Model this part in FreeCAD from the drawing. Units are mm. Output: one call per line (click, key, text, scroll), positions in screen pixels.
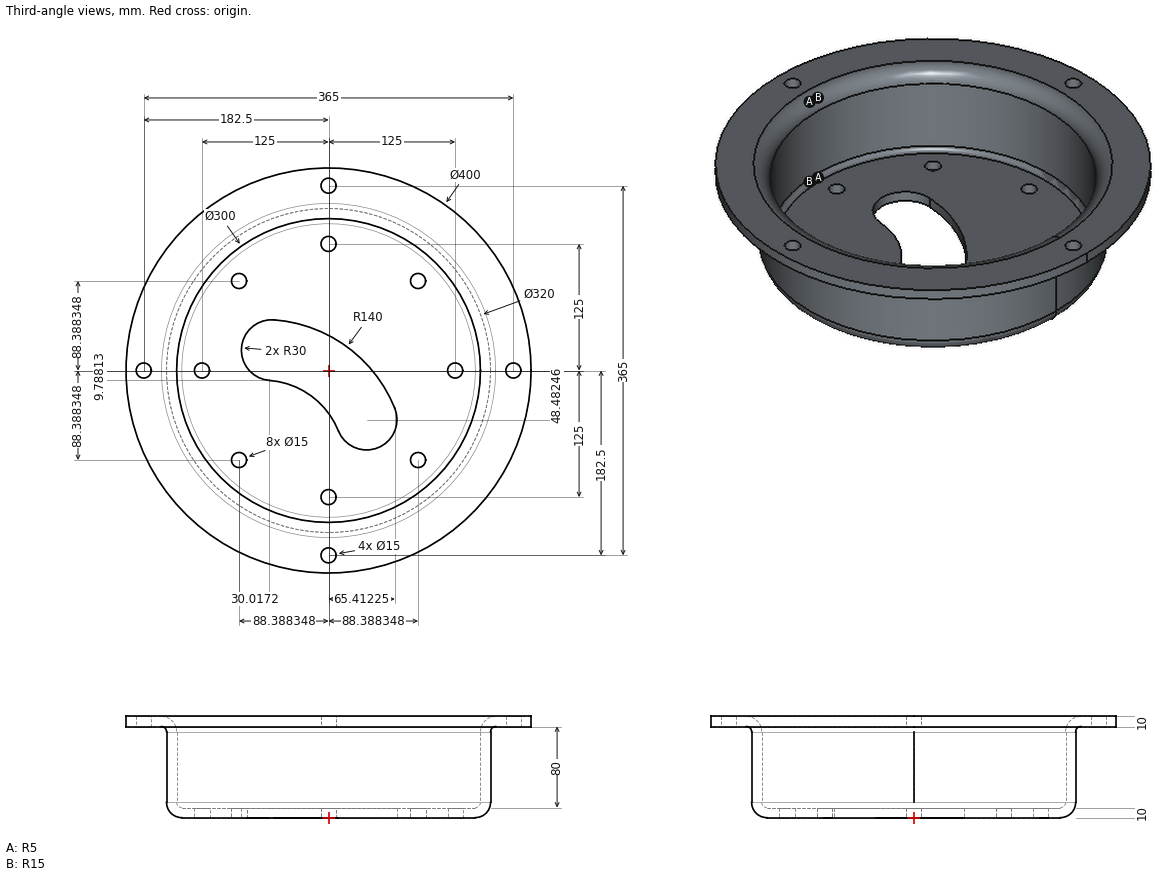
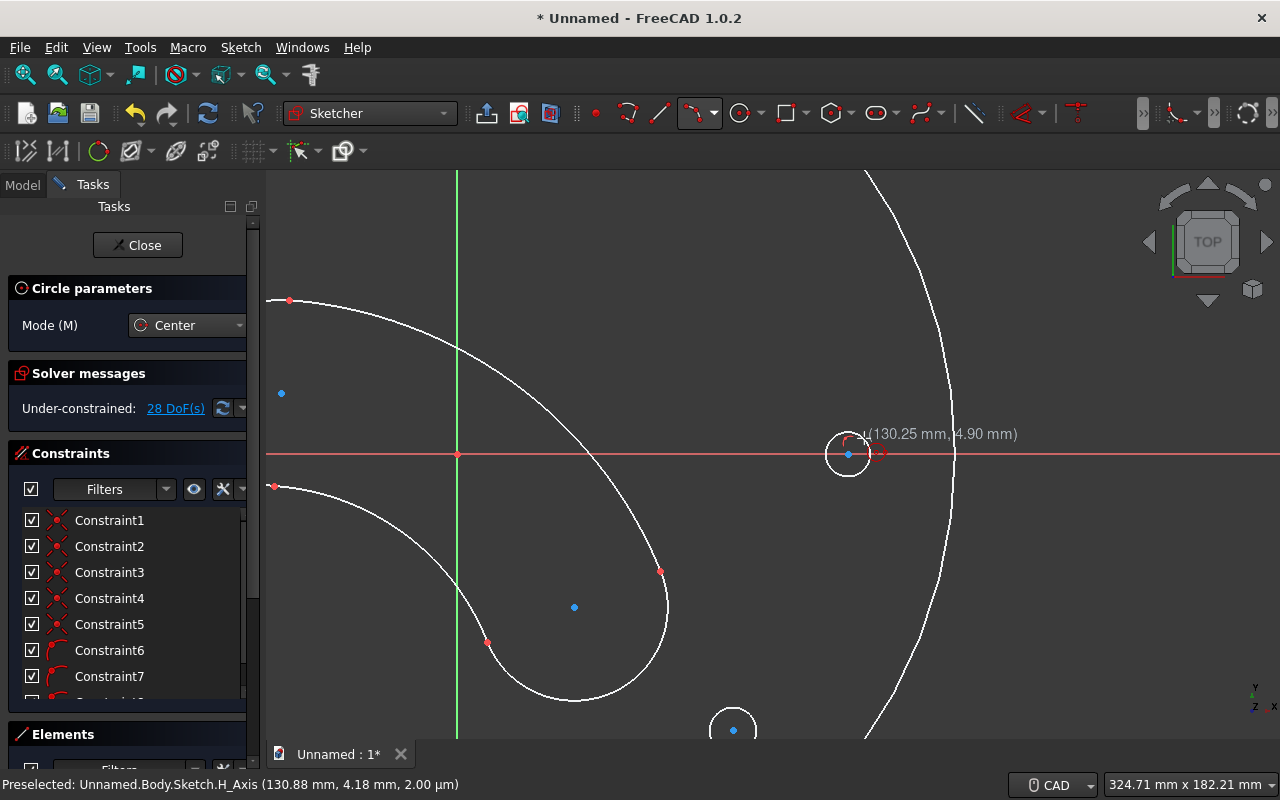
scroll(848, 455, down, 5)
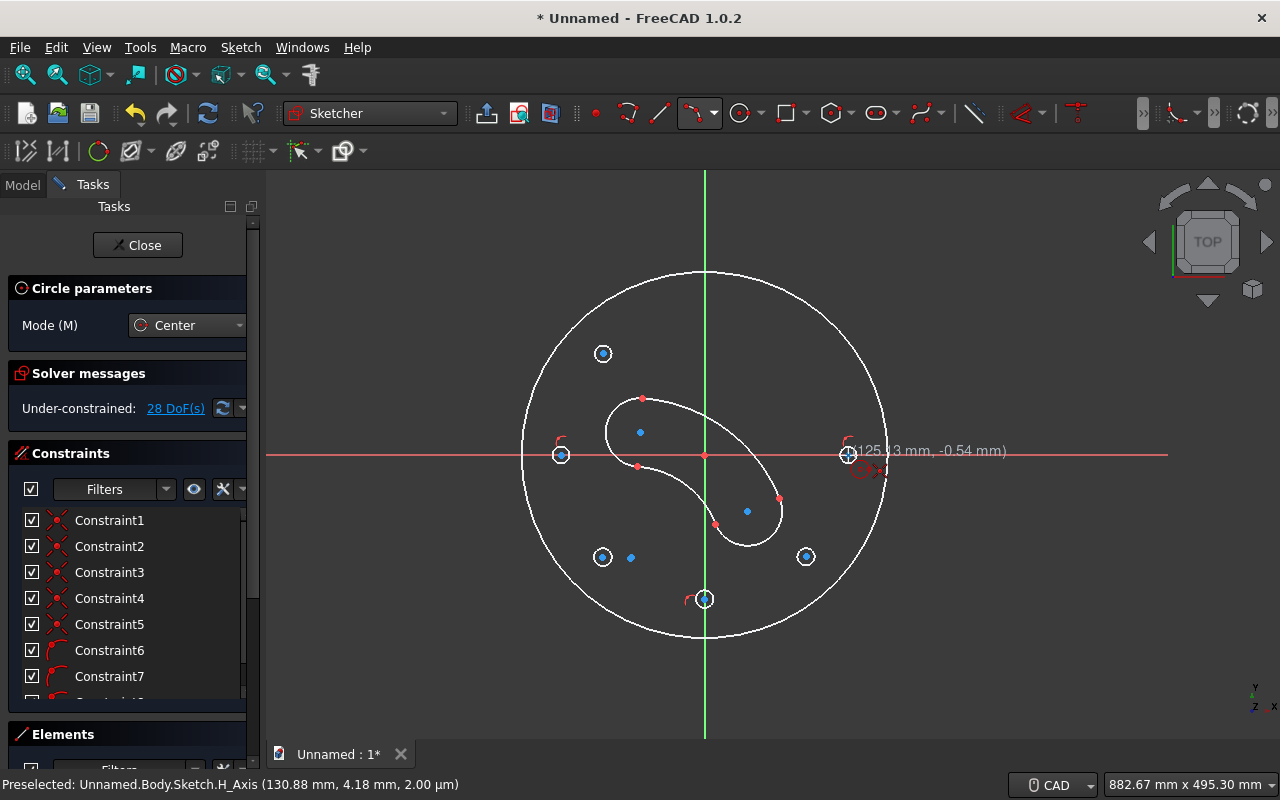
scroll(705, 311, up, 5)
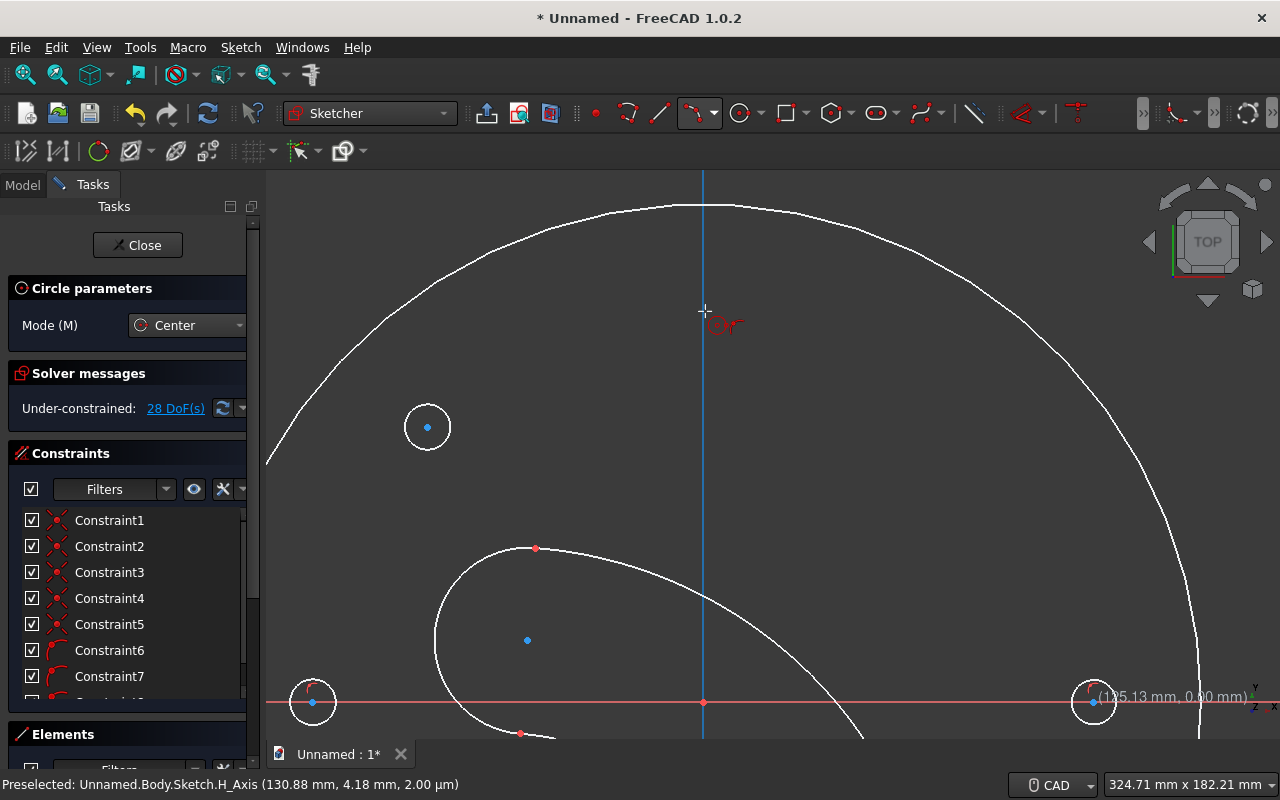
click(703, 312)
click(720, 295)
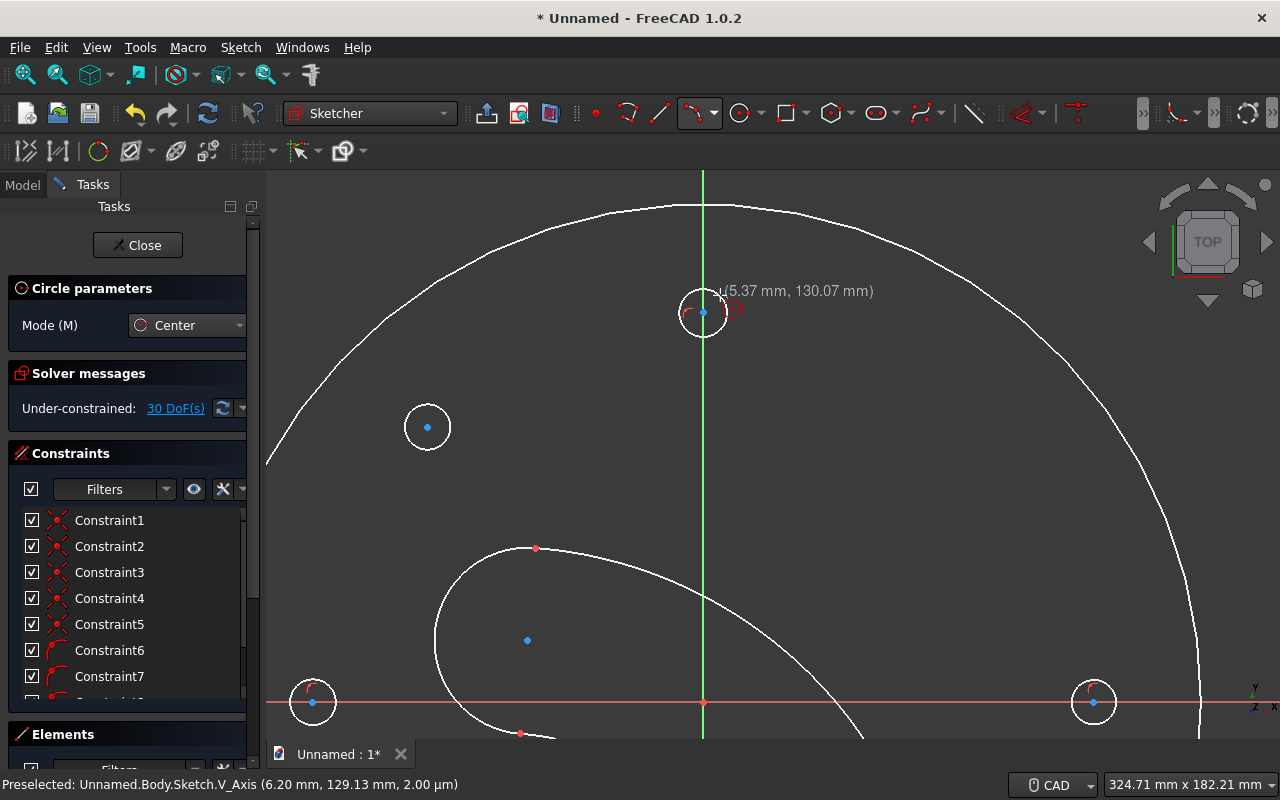
click(979, 426)
click(996, 410)
key(Escape)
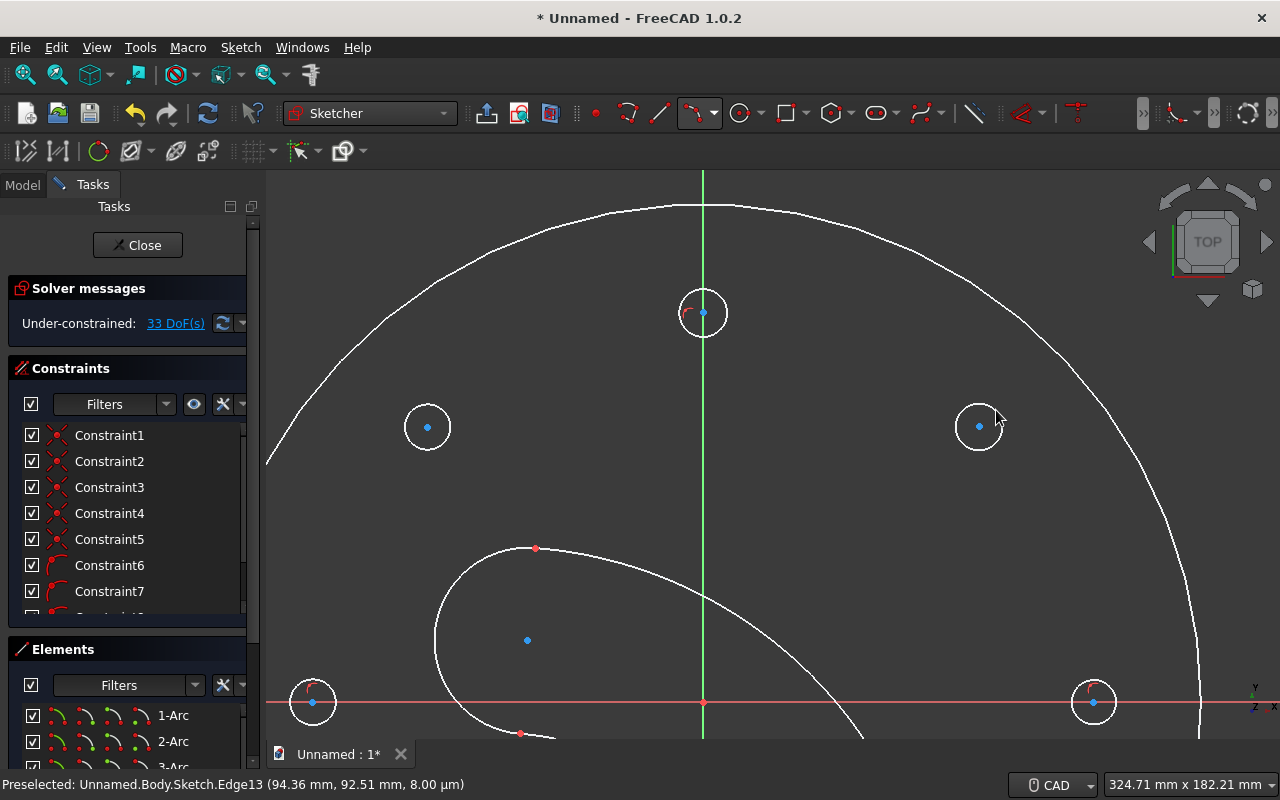
click(457, 580)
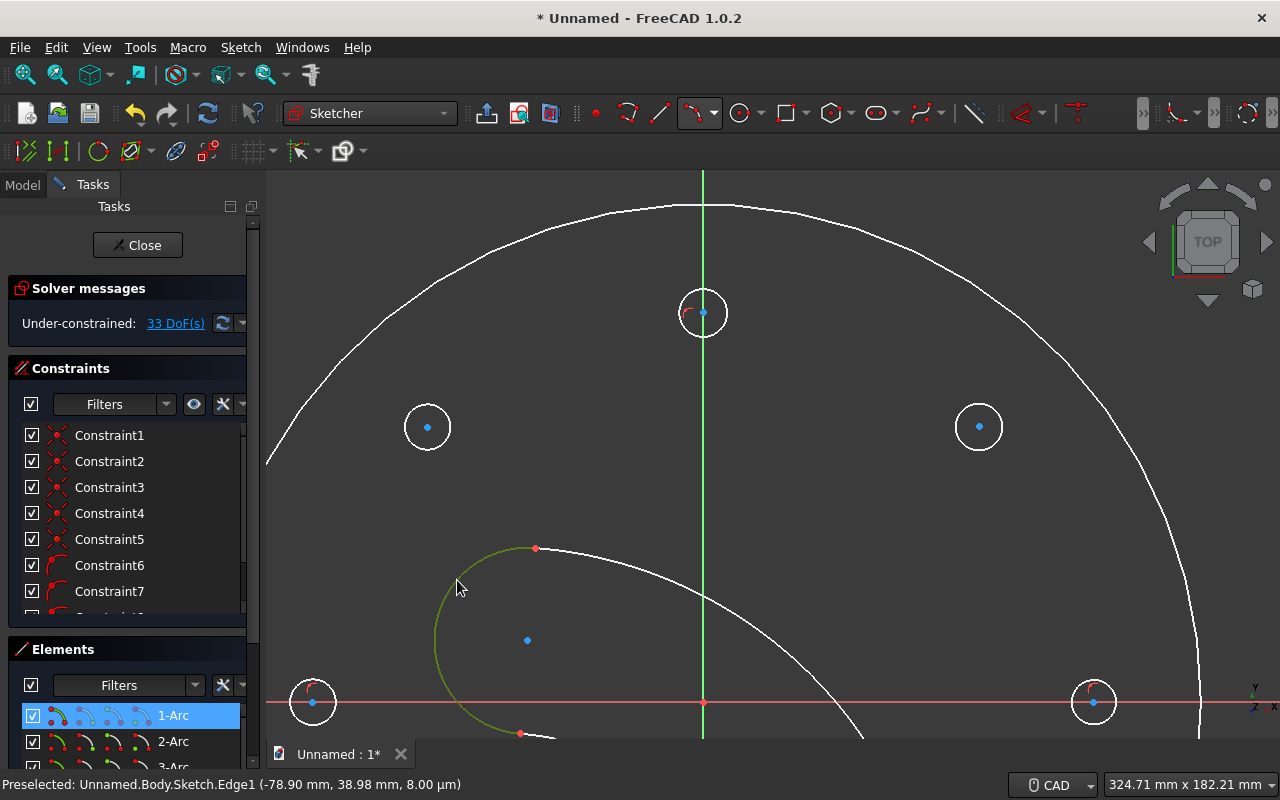
click(676, 583)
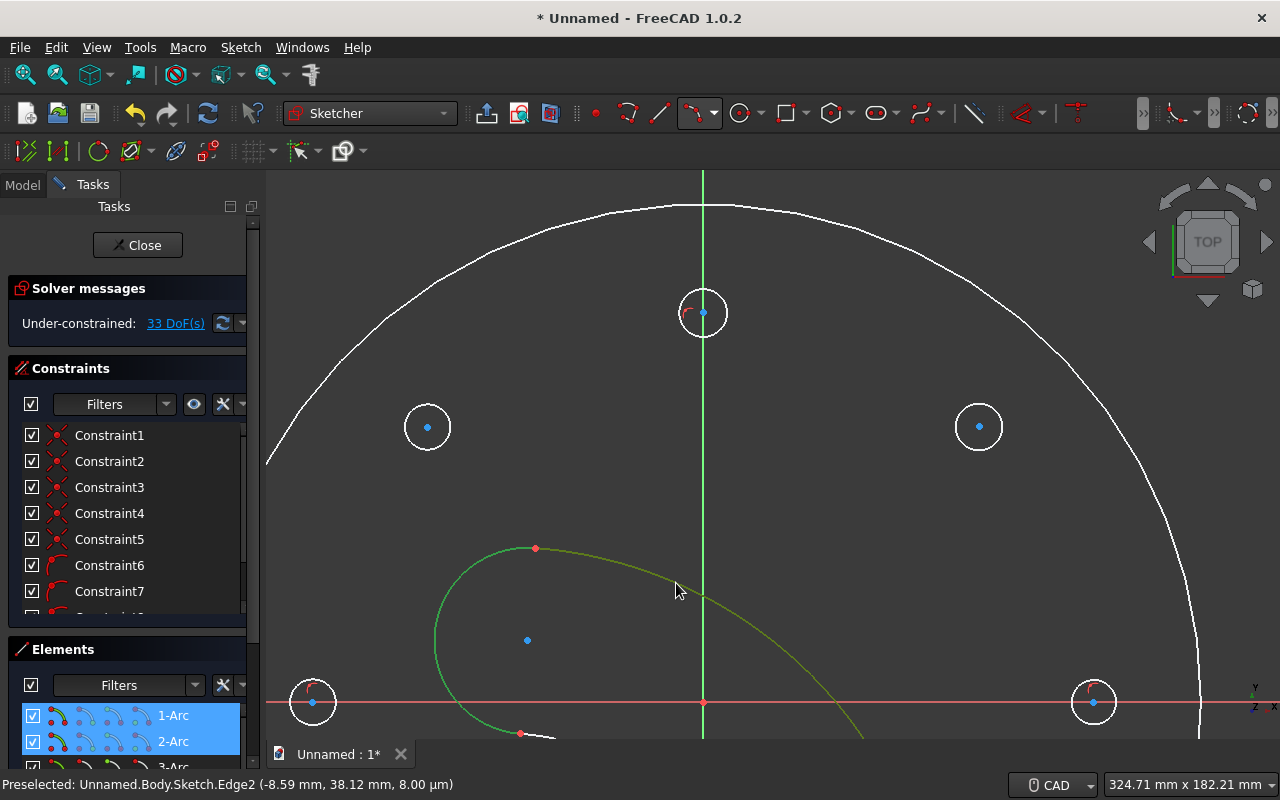
key(t)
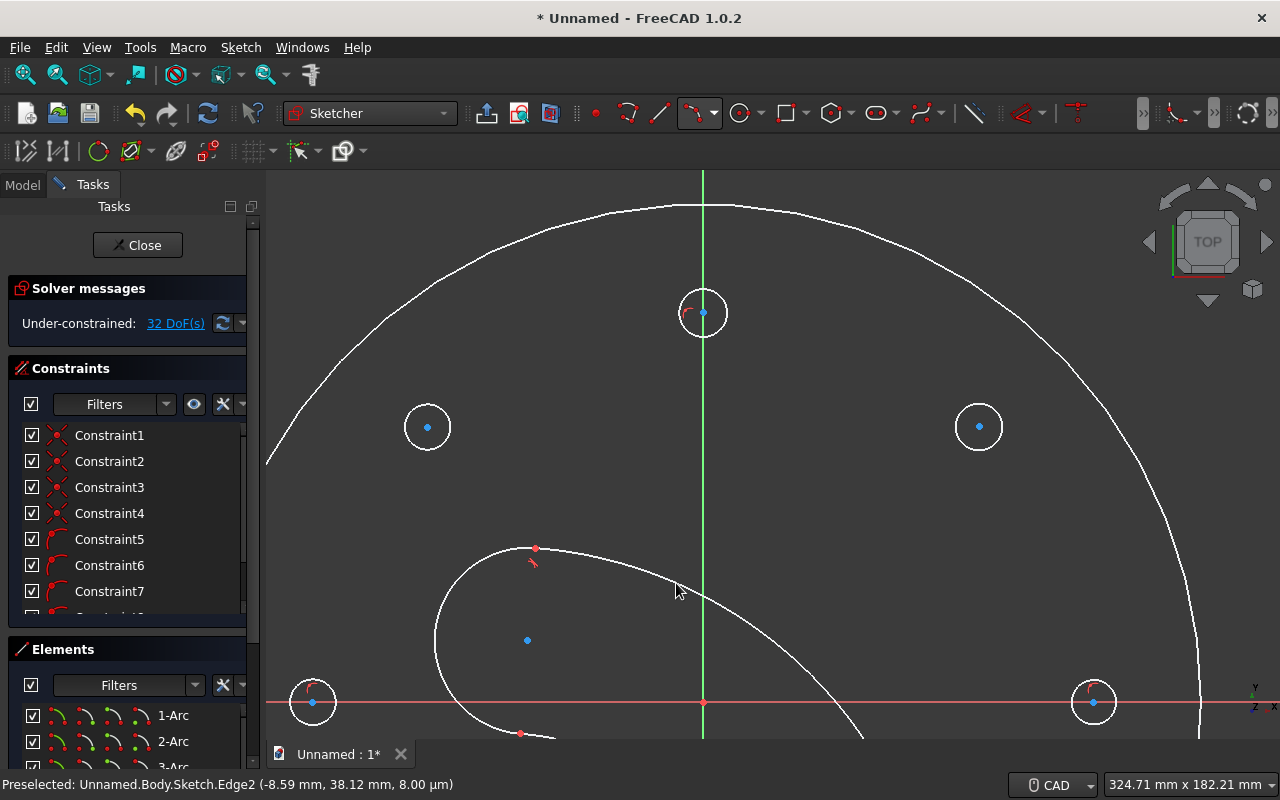
click(457, 581)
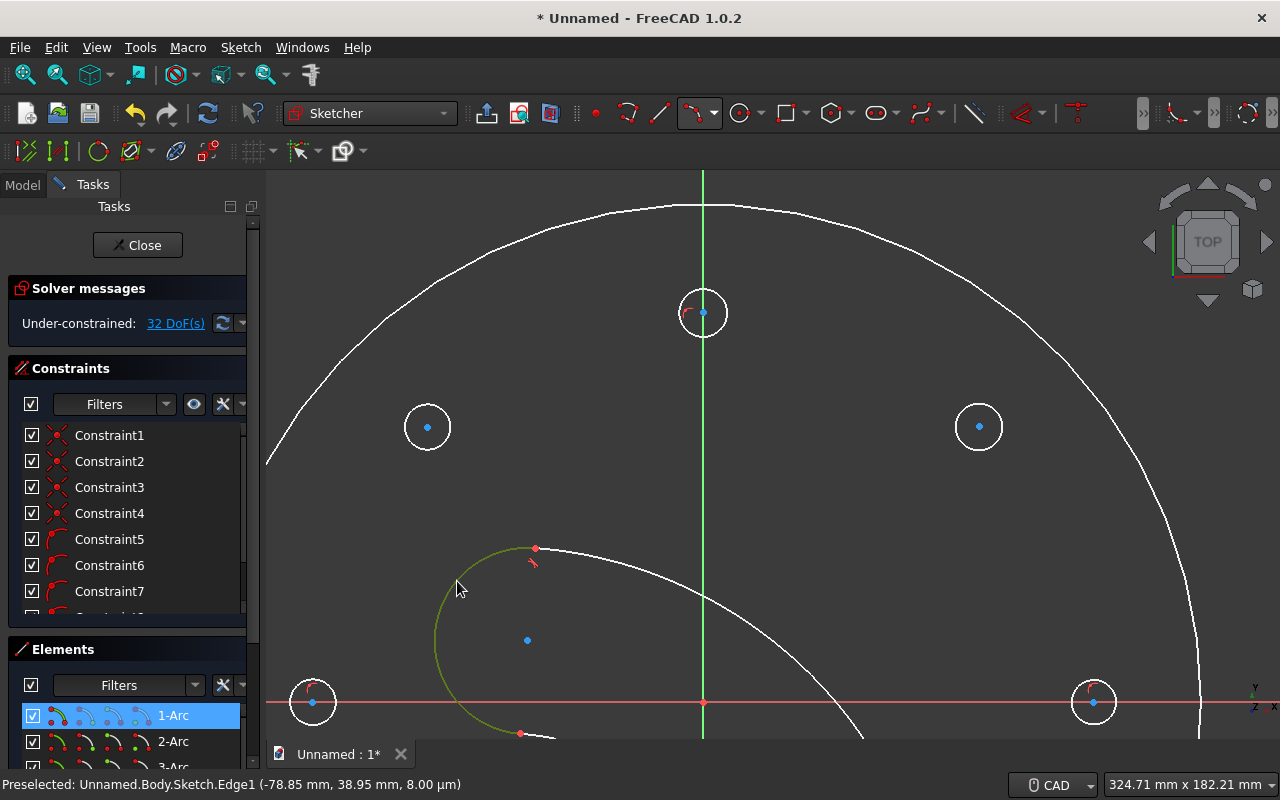
scroll(705, 310, down, 5)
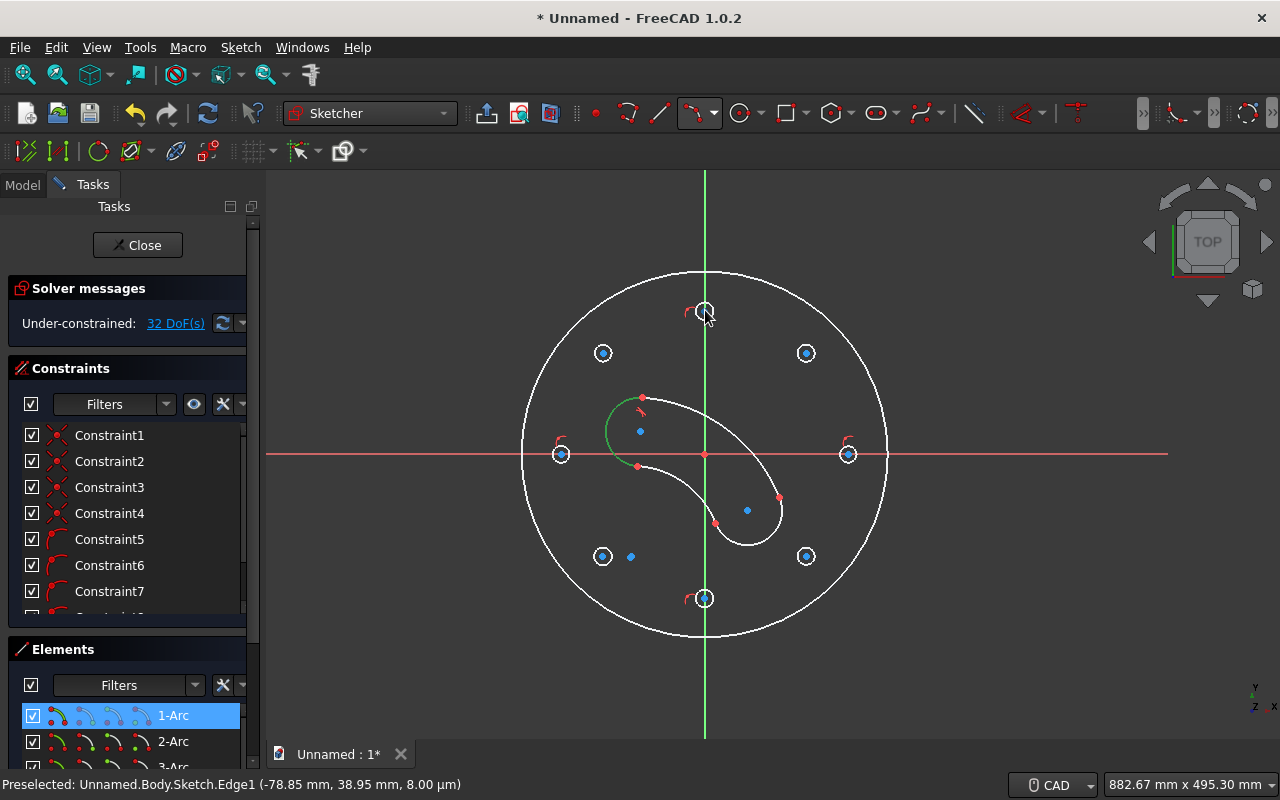
scroll(700, 497, up, 6)